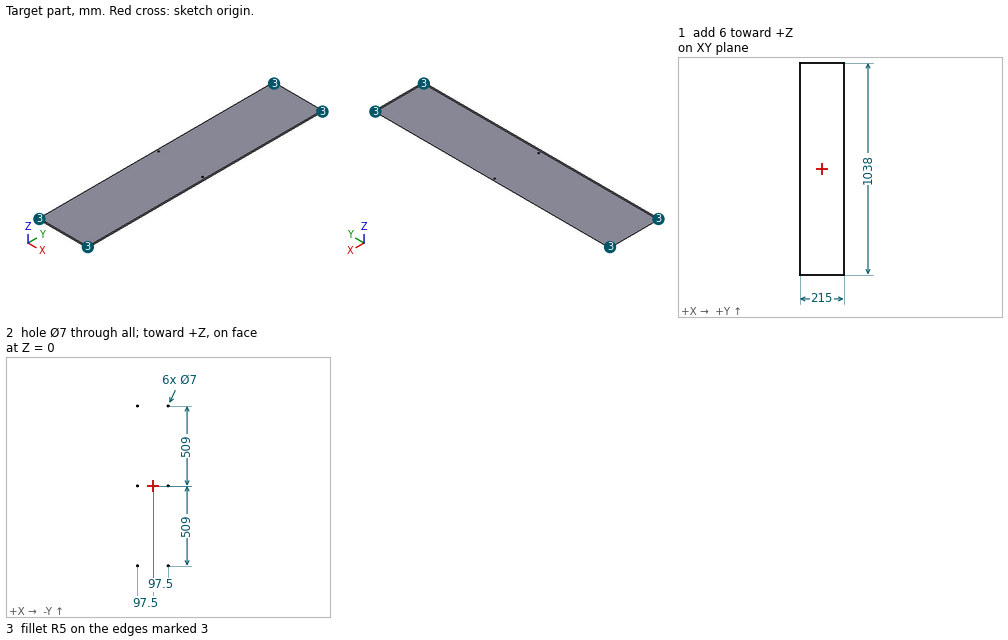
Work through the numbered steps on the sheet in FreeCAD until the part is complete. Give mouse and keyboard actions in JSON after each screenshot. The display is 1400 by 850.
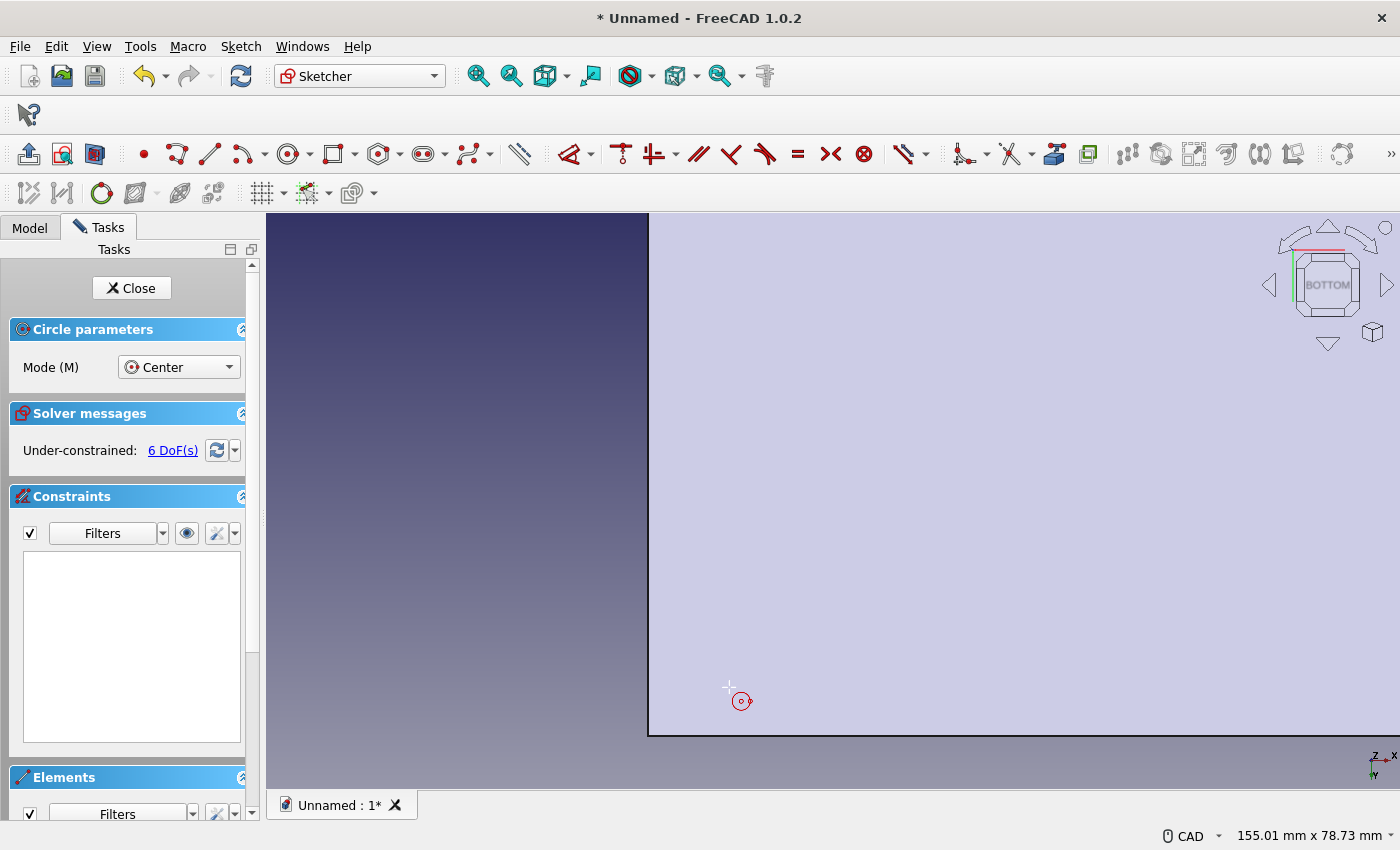
{"action": "scroll", "coordinate": [729, 688], "scroll_direction": "down", "scroll_amount": 15}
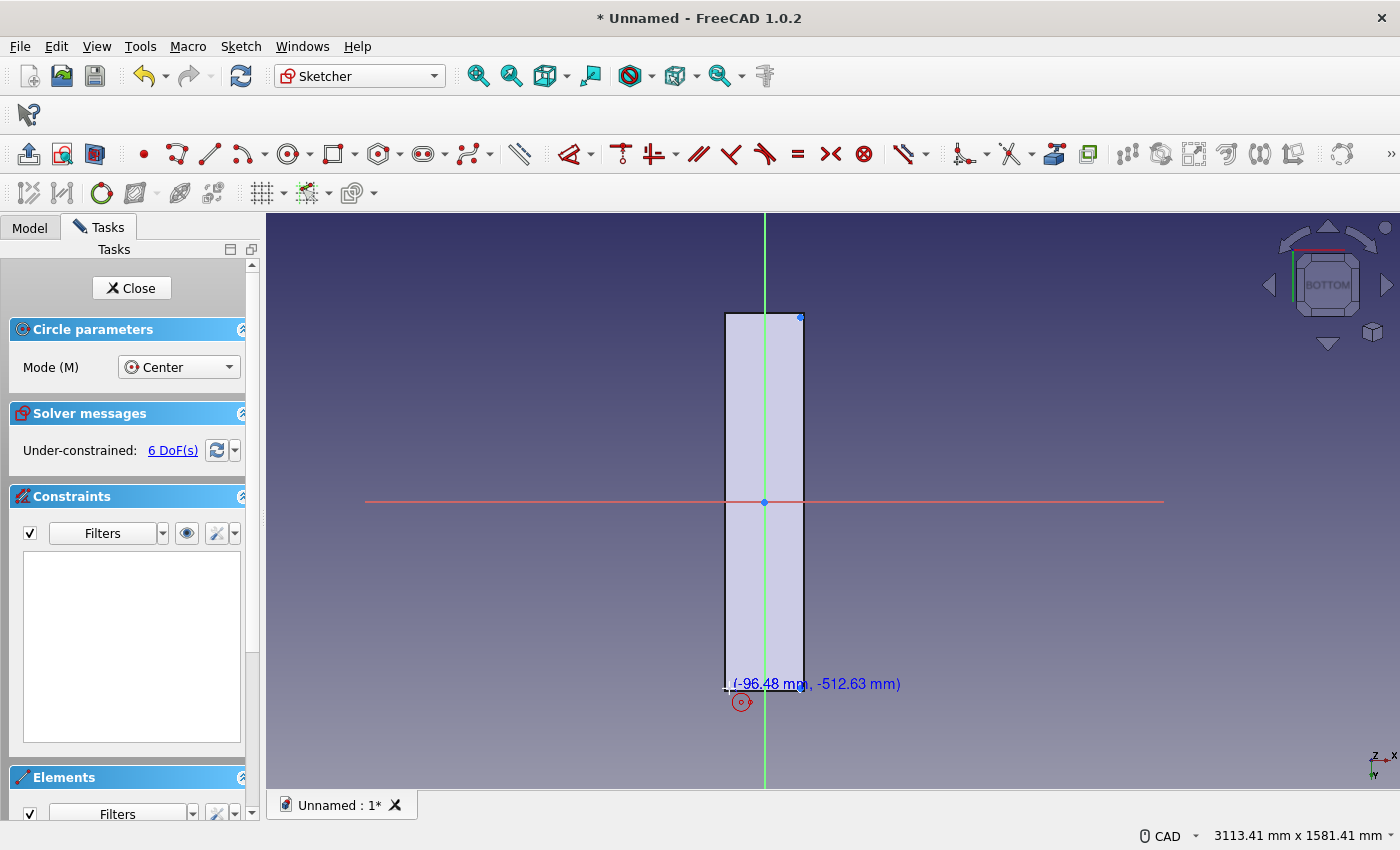
{"action": "left_click", "coordinate": [729, 688]}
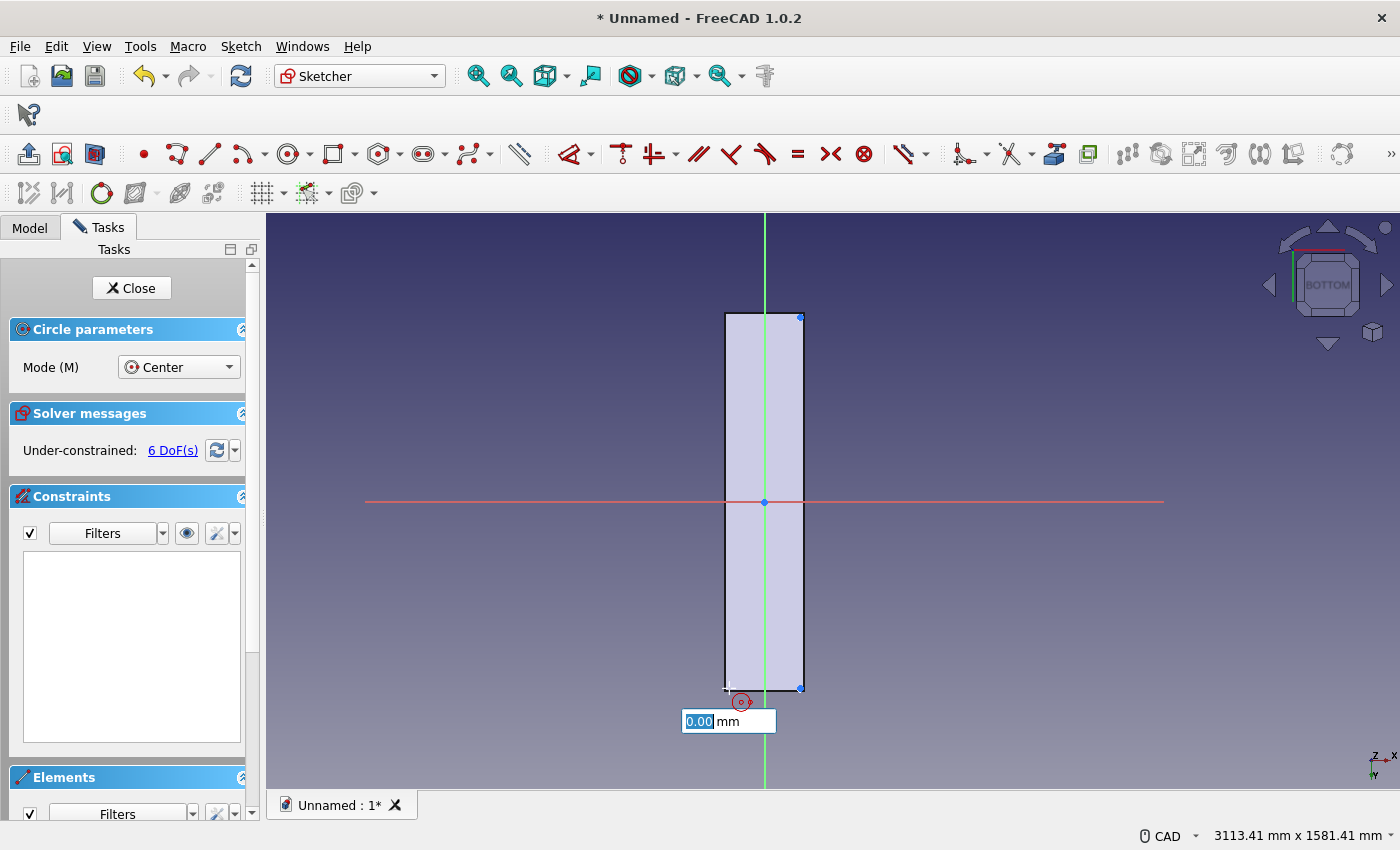
{"action": "scroll", "coordinate": [730, 687], "scroll_direction": "up", "scroll_amount": 13}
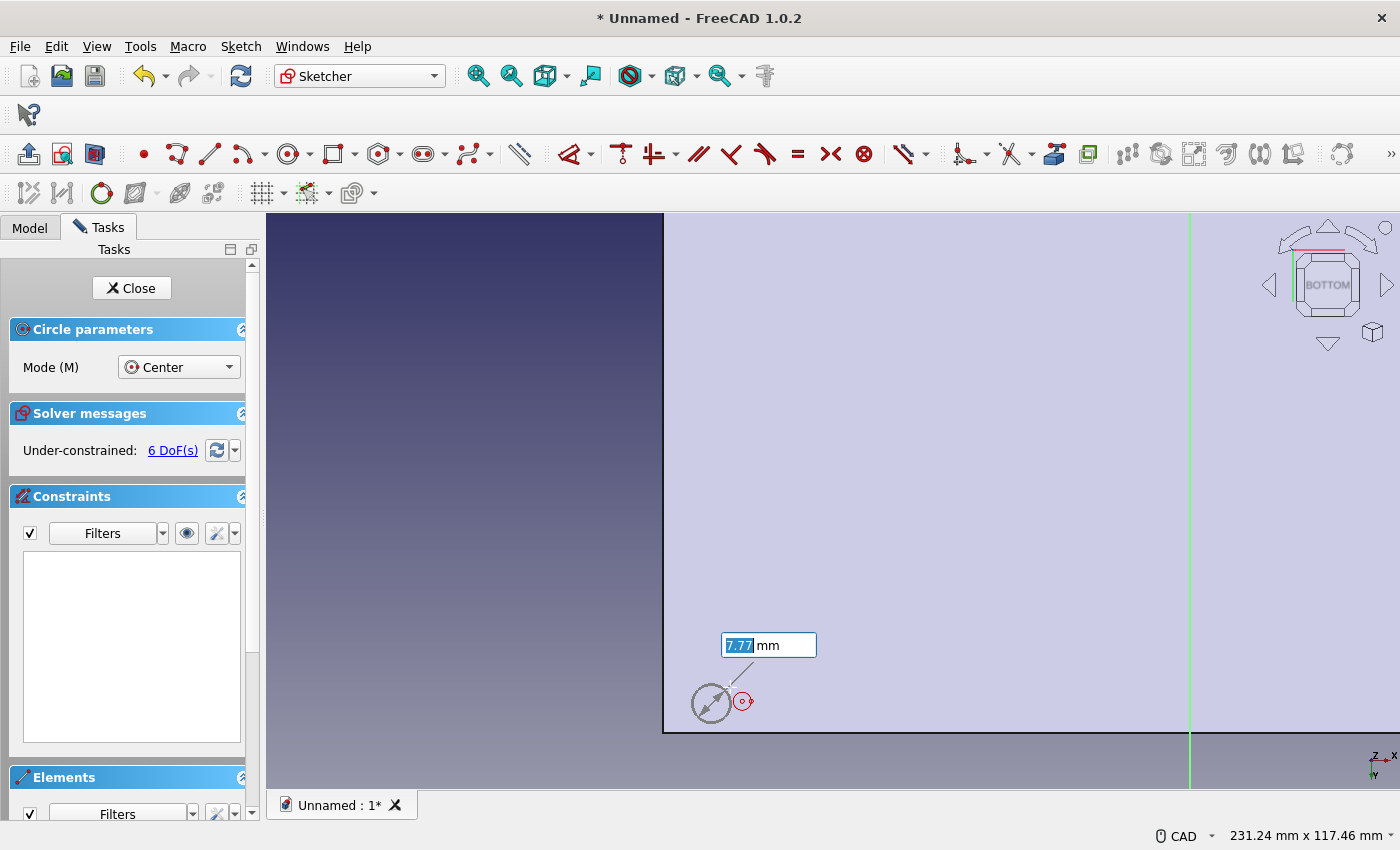
{"action": "left_click", "coordinate": [724, 671]}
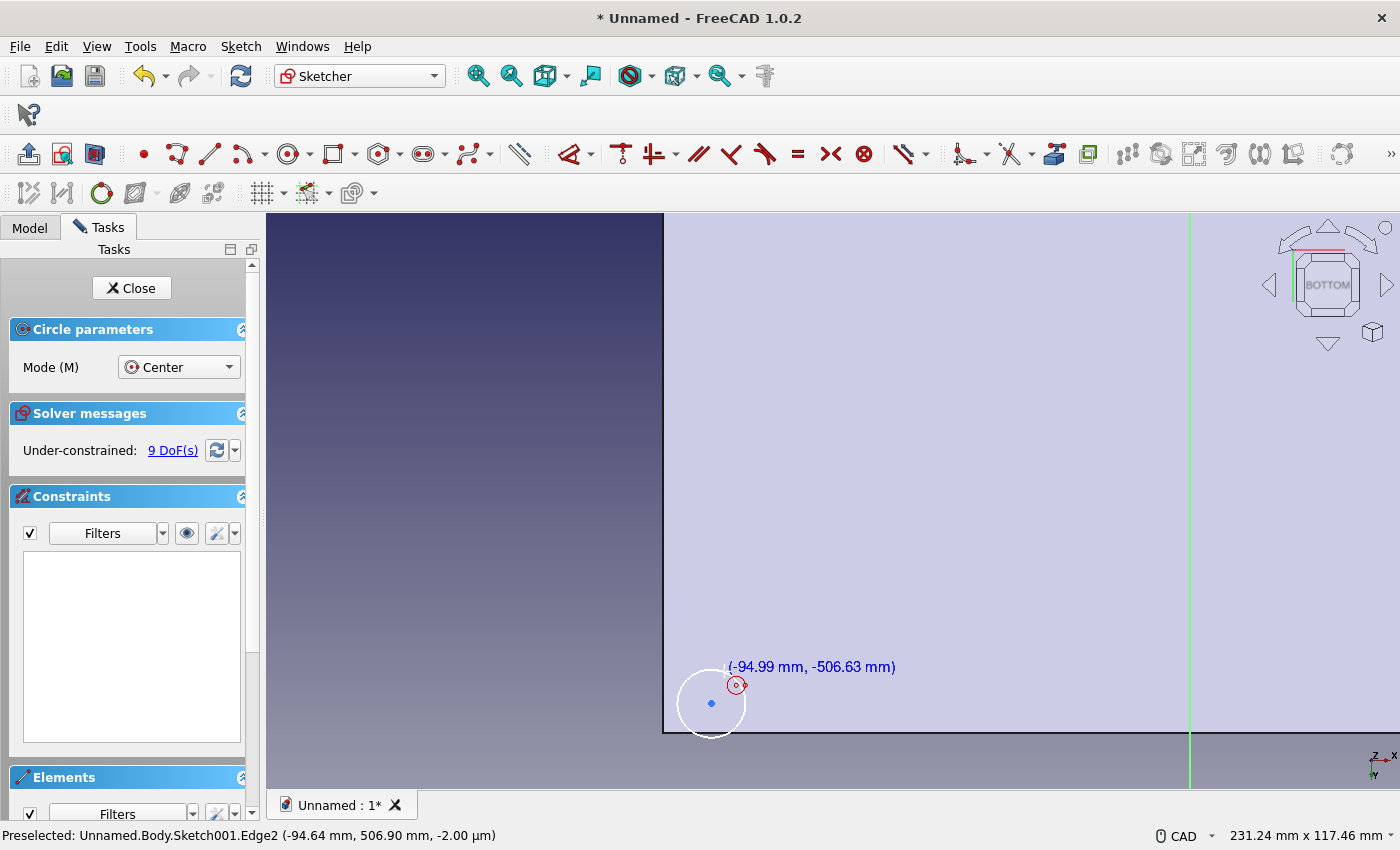
{"action": "scroll", "coordinate": [730, 687], "scroll_direction": "down", "scroll_amount": 13}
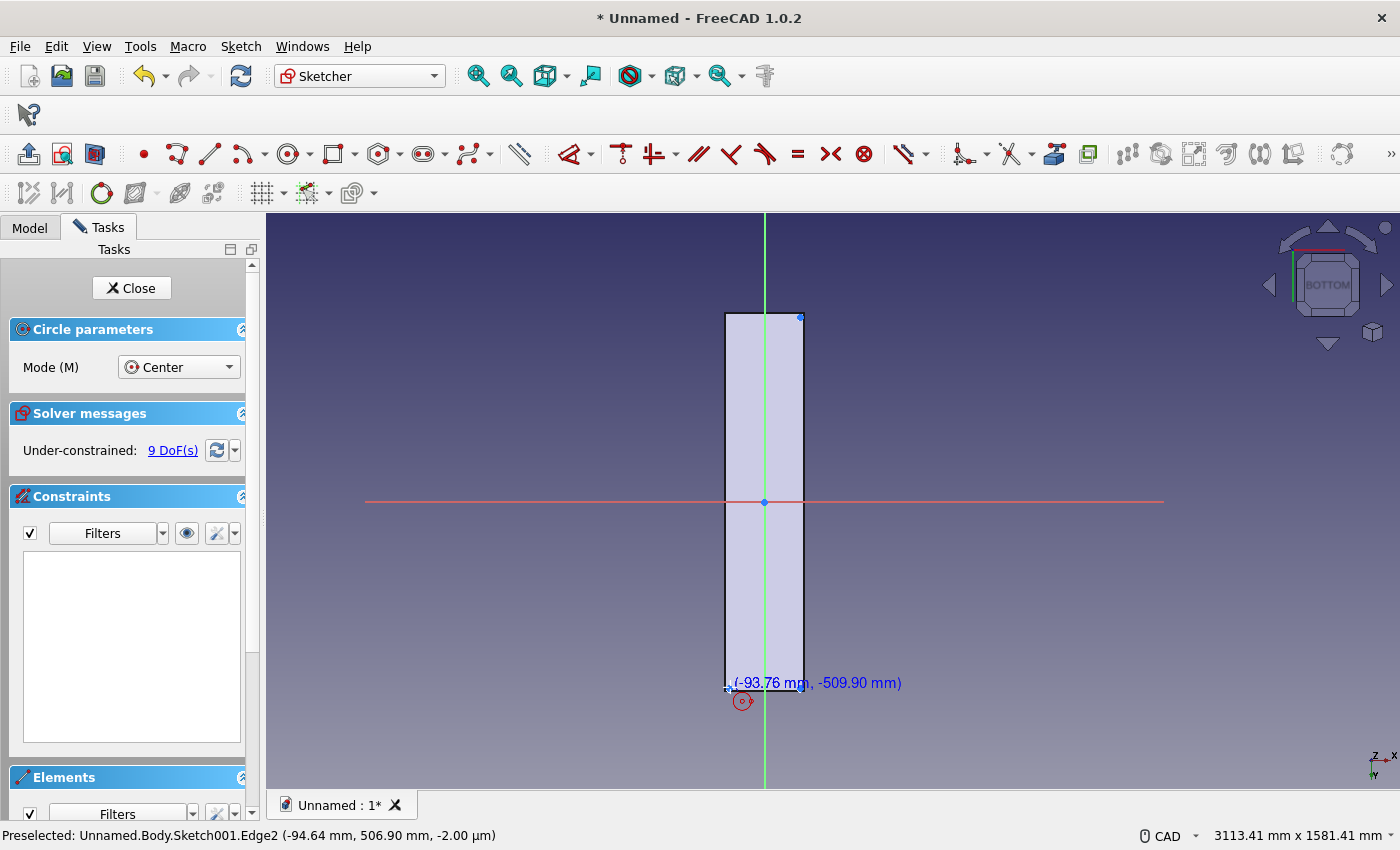
{"action": "scroll", "coordinate": [729, 317], "scroll_direction": "up", "scroll_amount": 15}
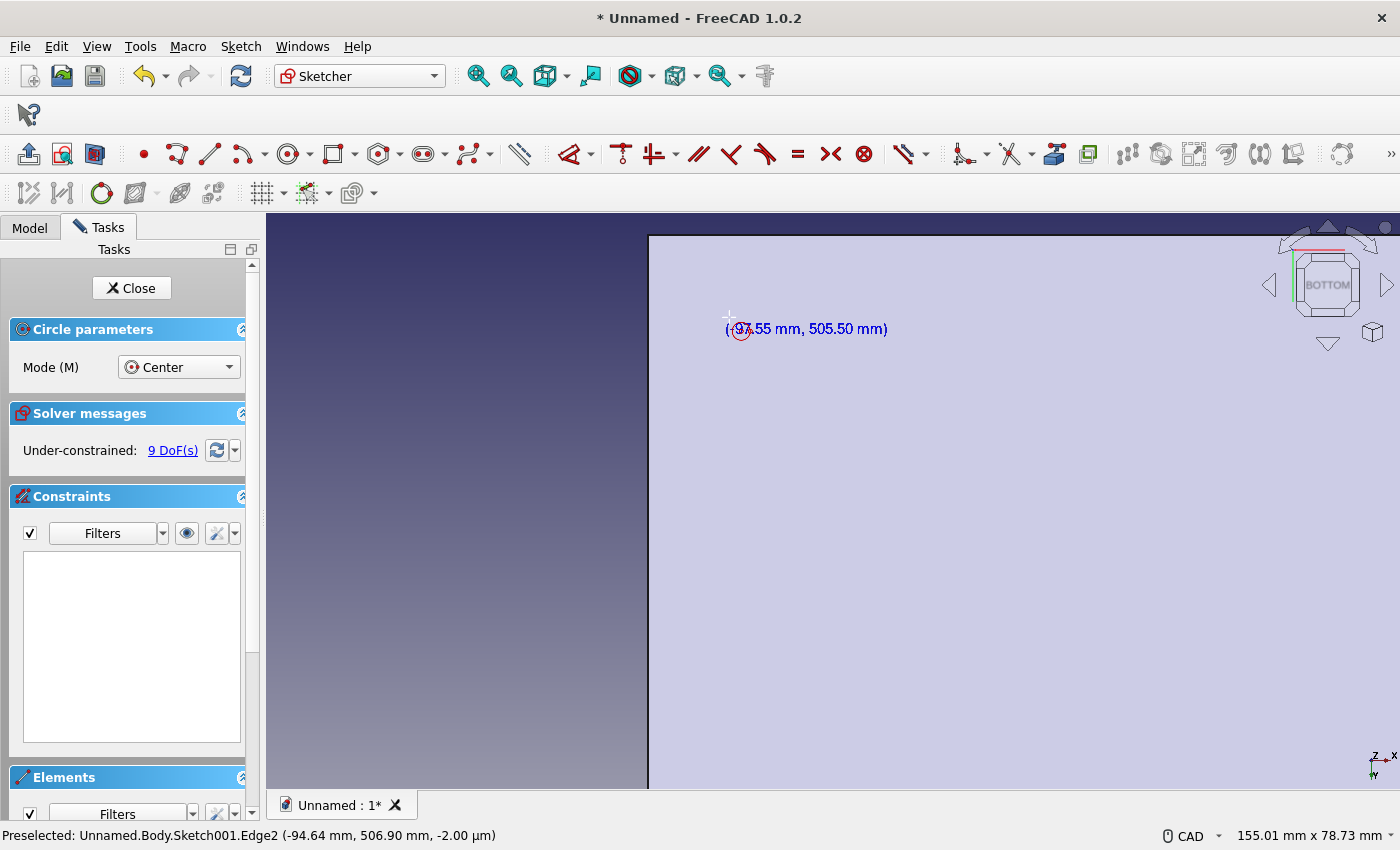
{"action": "scroll", "coordinate": [729, 316], "scroll_direction": "down", "scroll_amount": 15}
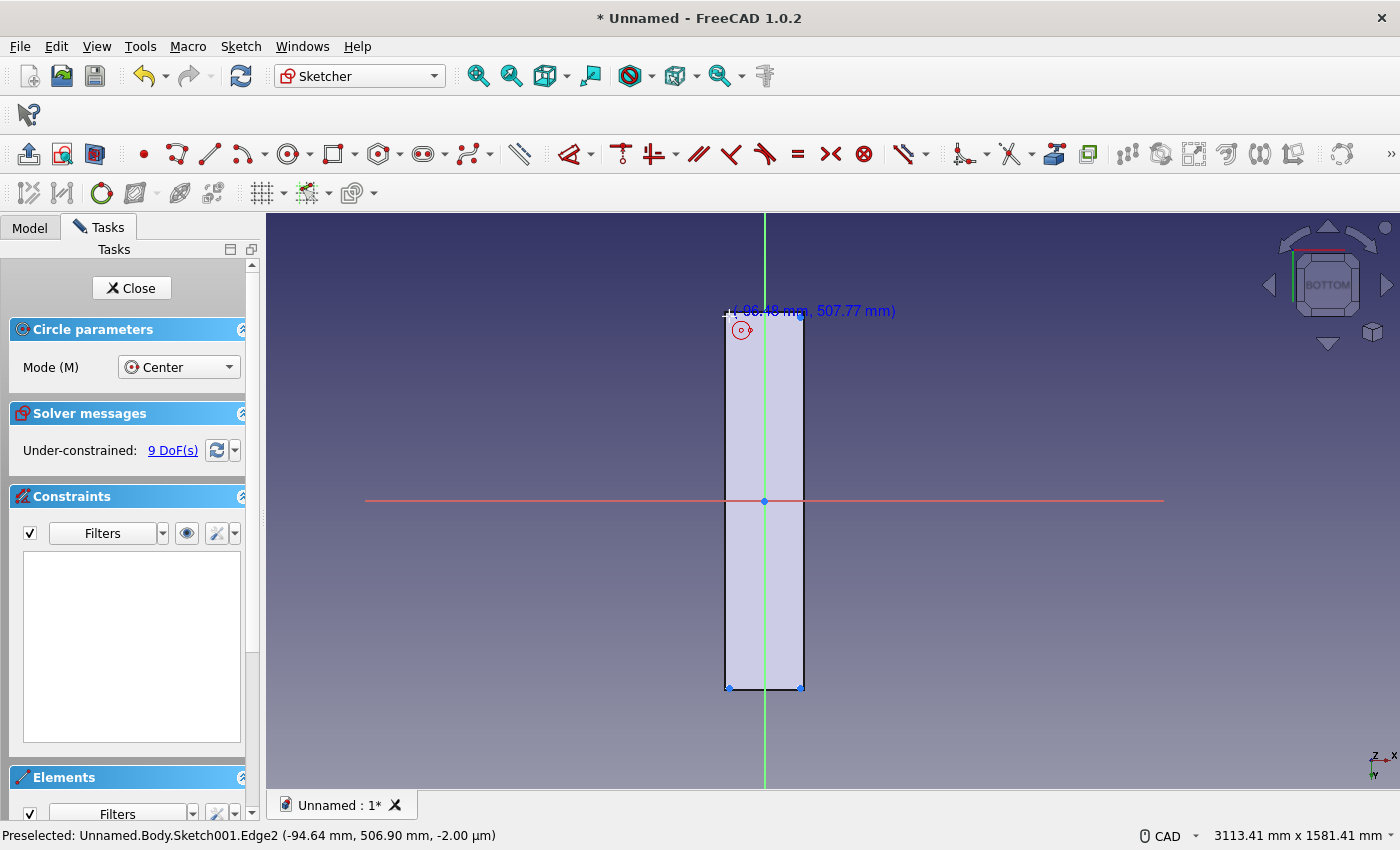
{"action": "left_click", "coordinate": [729, 316]}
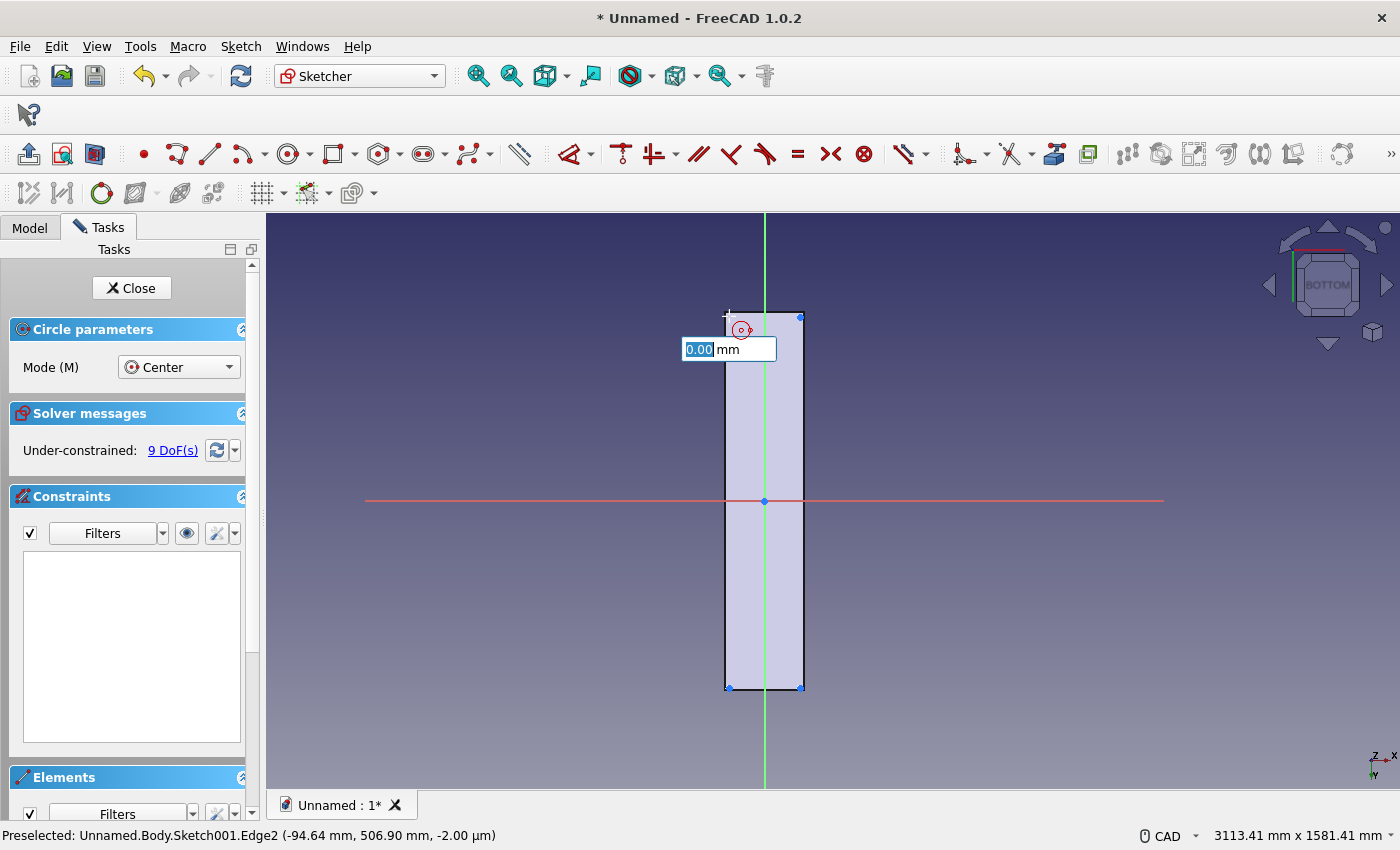
{"action": "scroll", "coordinate": [730, 315], "scroll_direction": "up", "scroll_amount": 13}